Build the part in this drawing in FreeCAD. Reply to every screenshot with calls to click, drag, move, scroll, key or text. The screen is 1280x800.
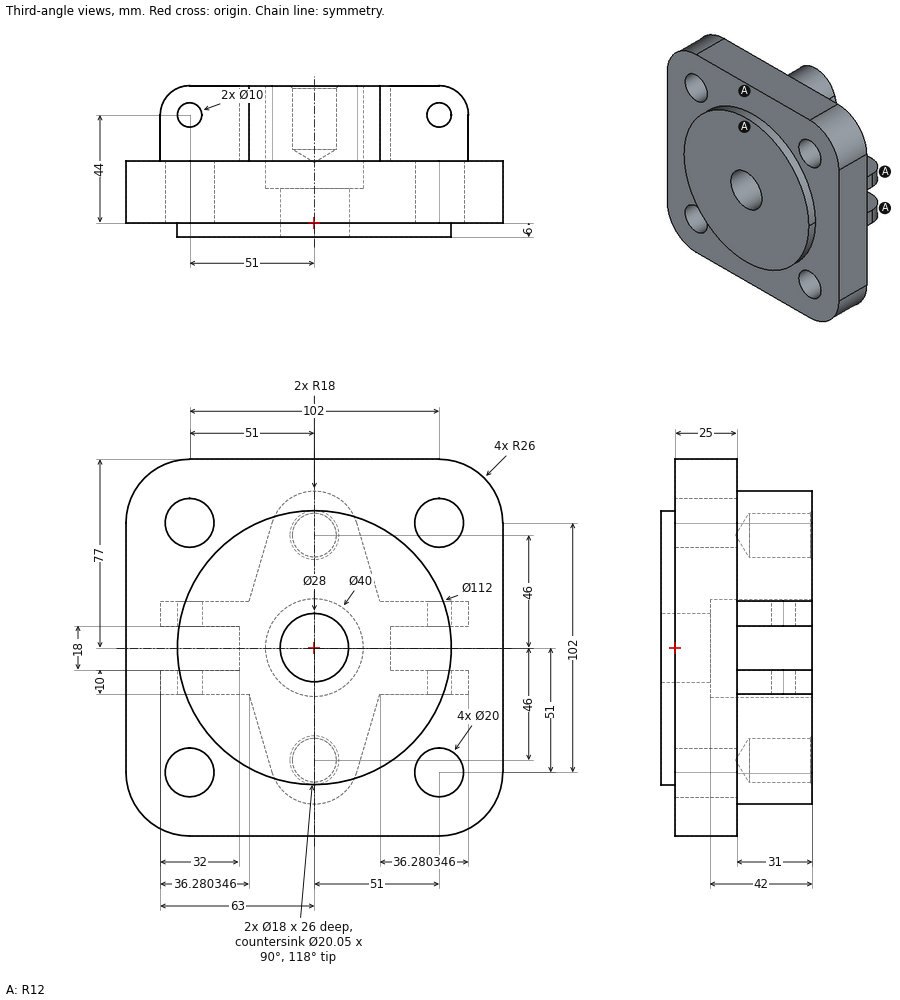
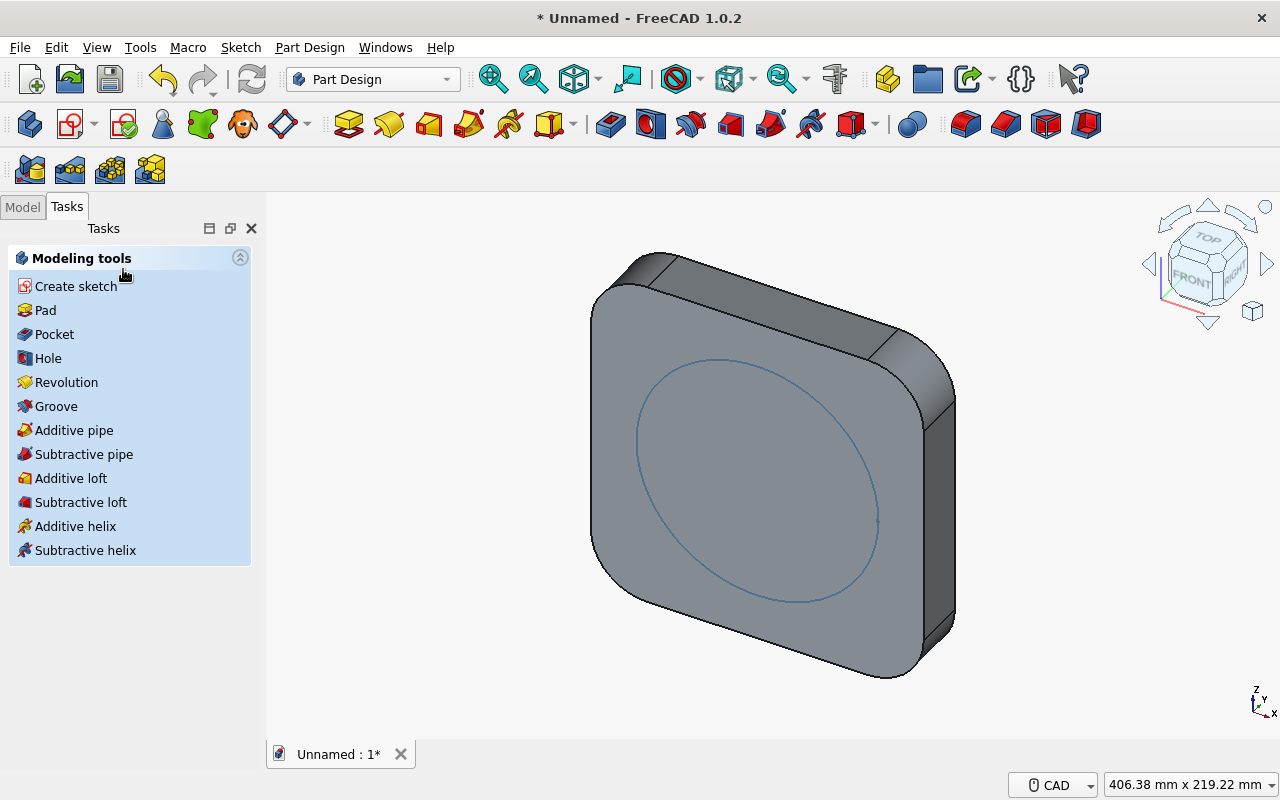
click(350, 124)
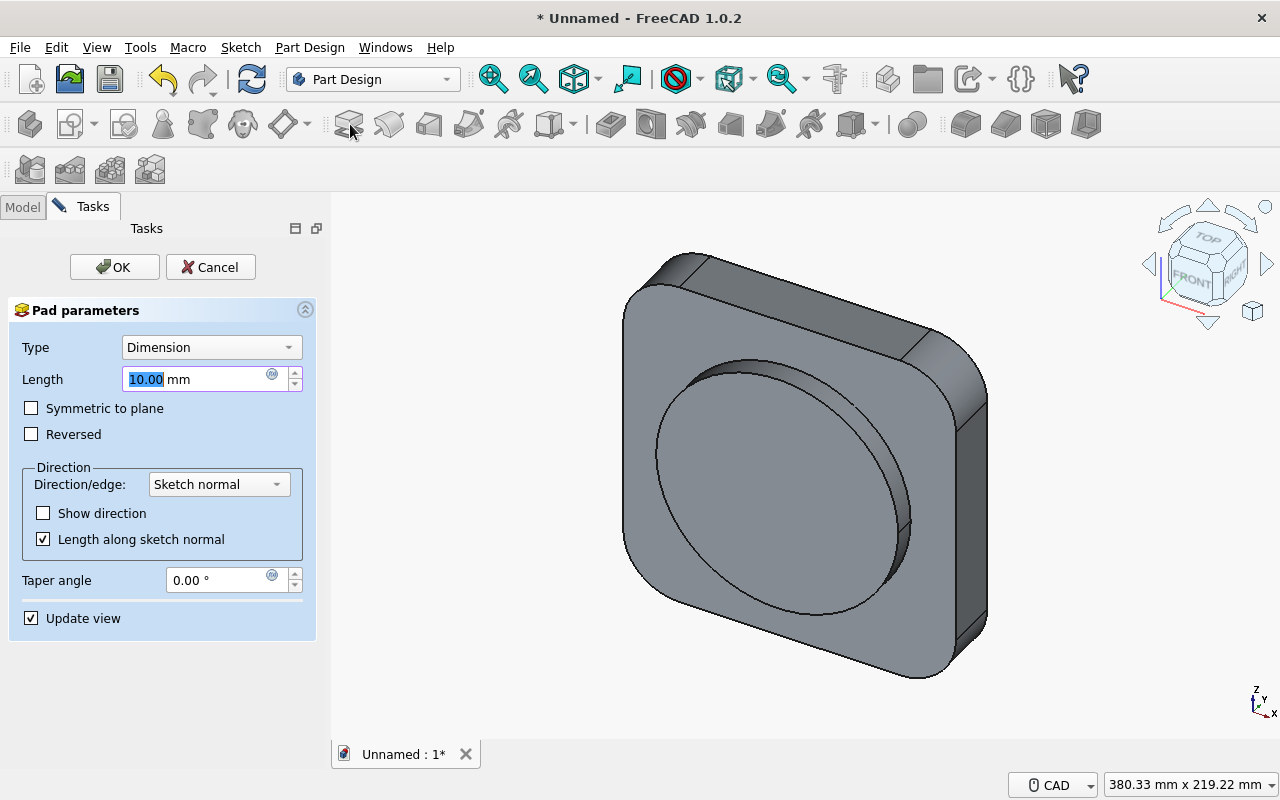
text(6)
key(Tab)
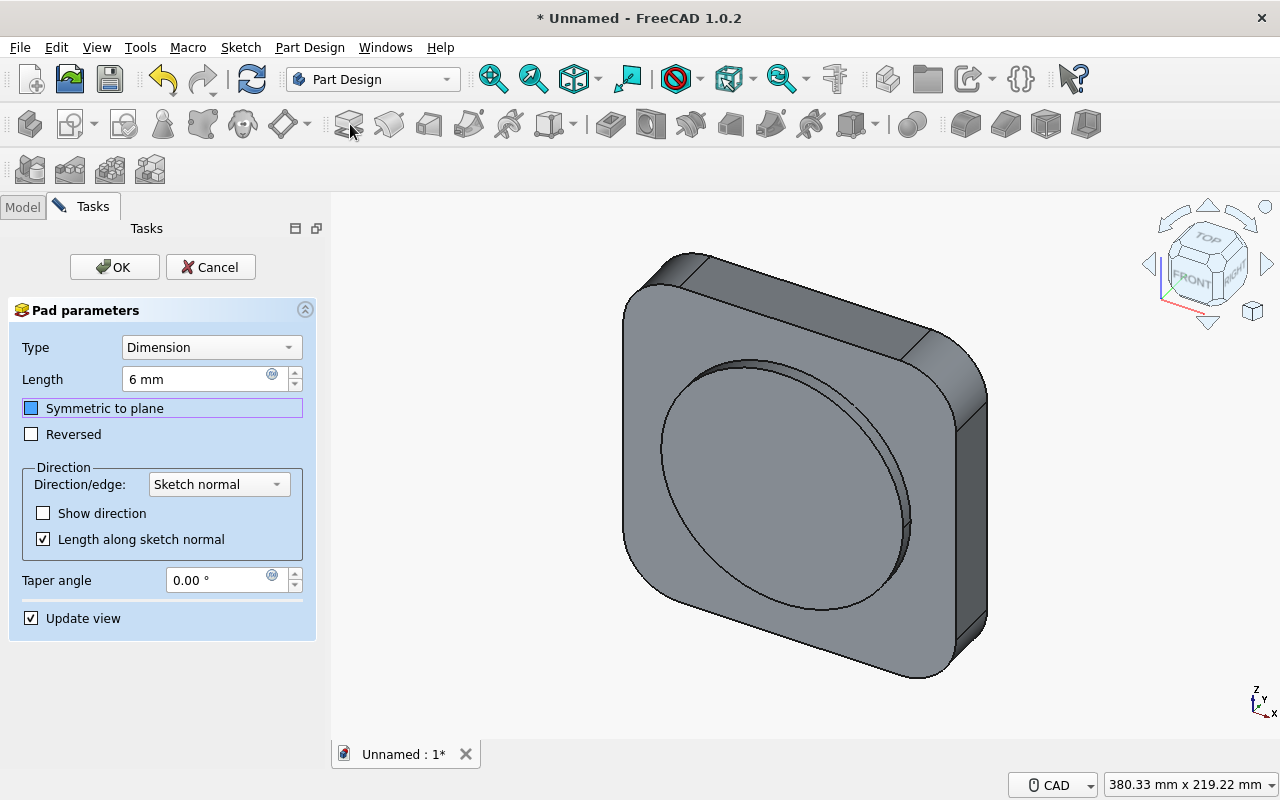
click(115, 267)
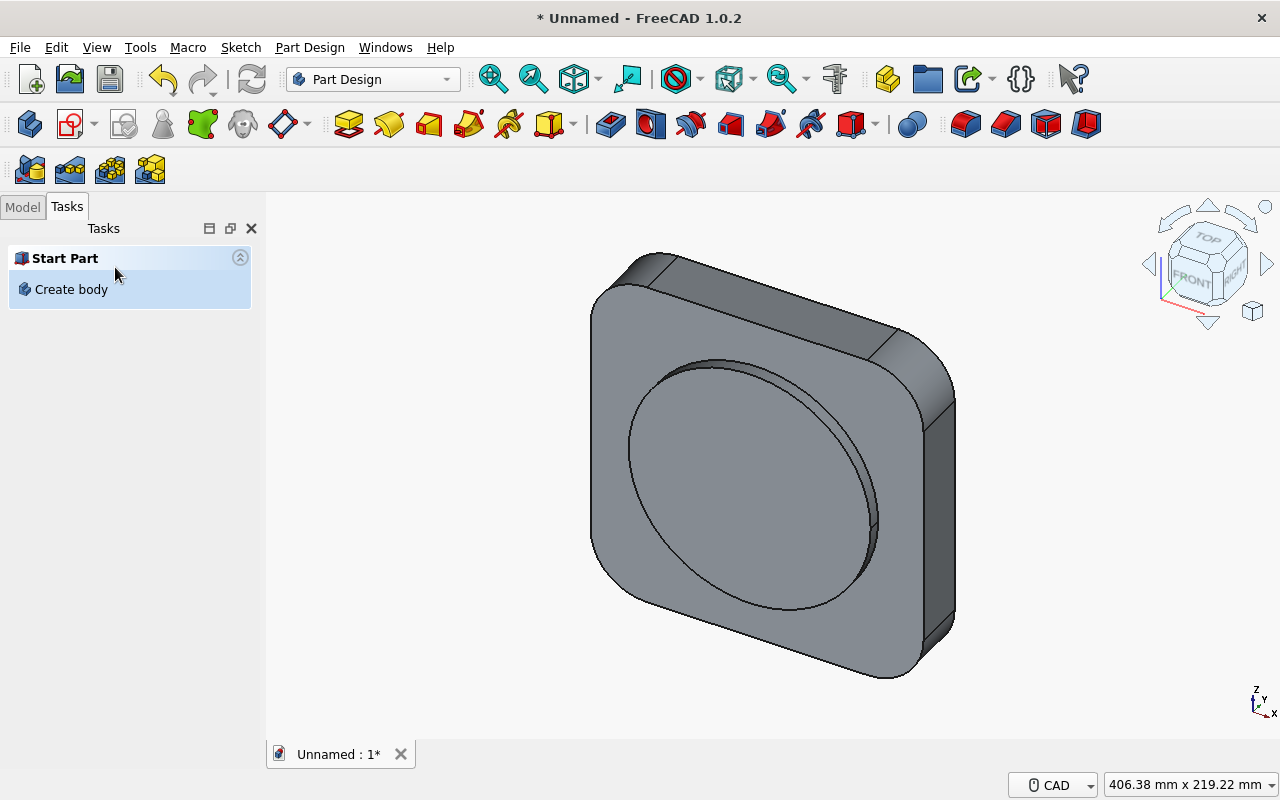
key(4)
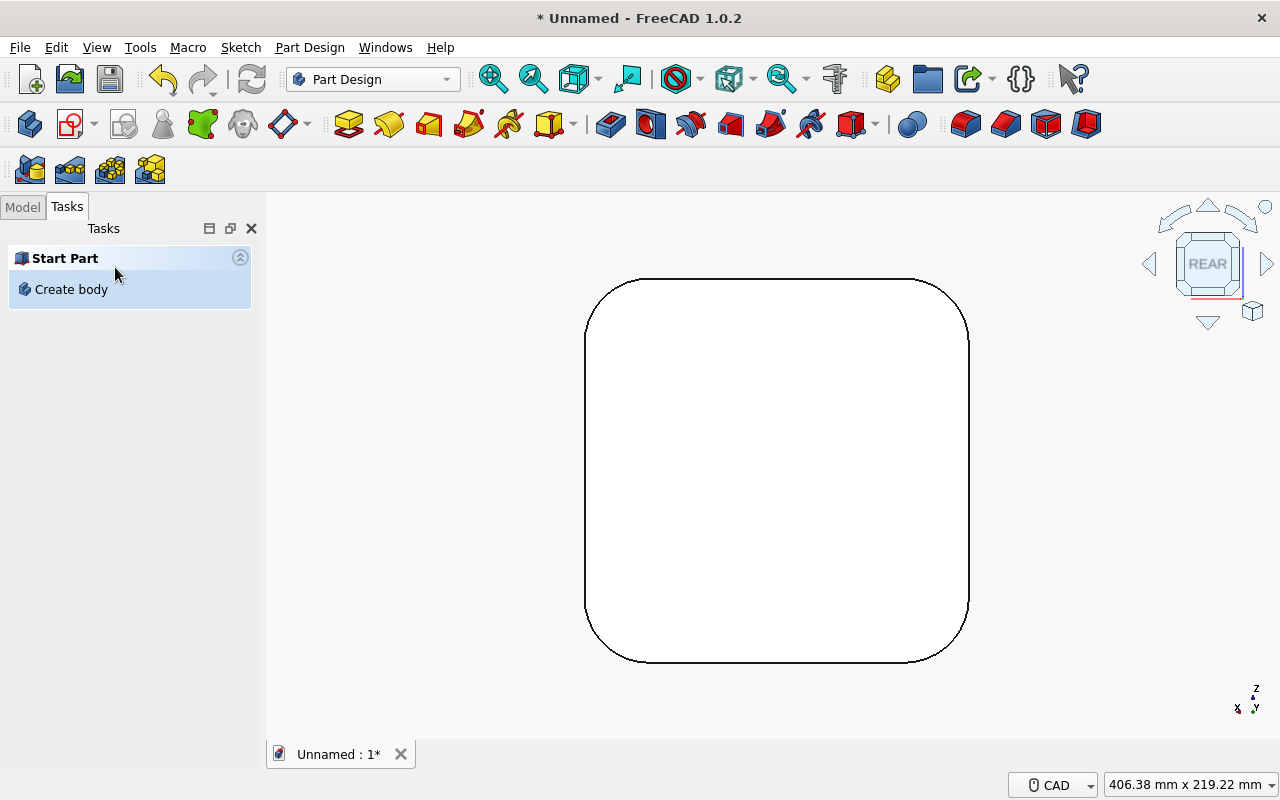
click(777, 470)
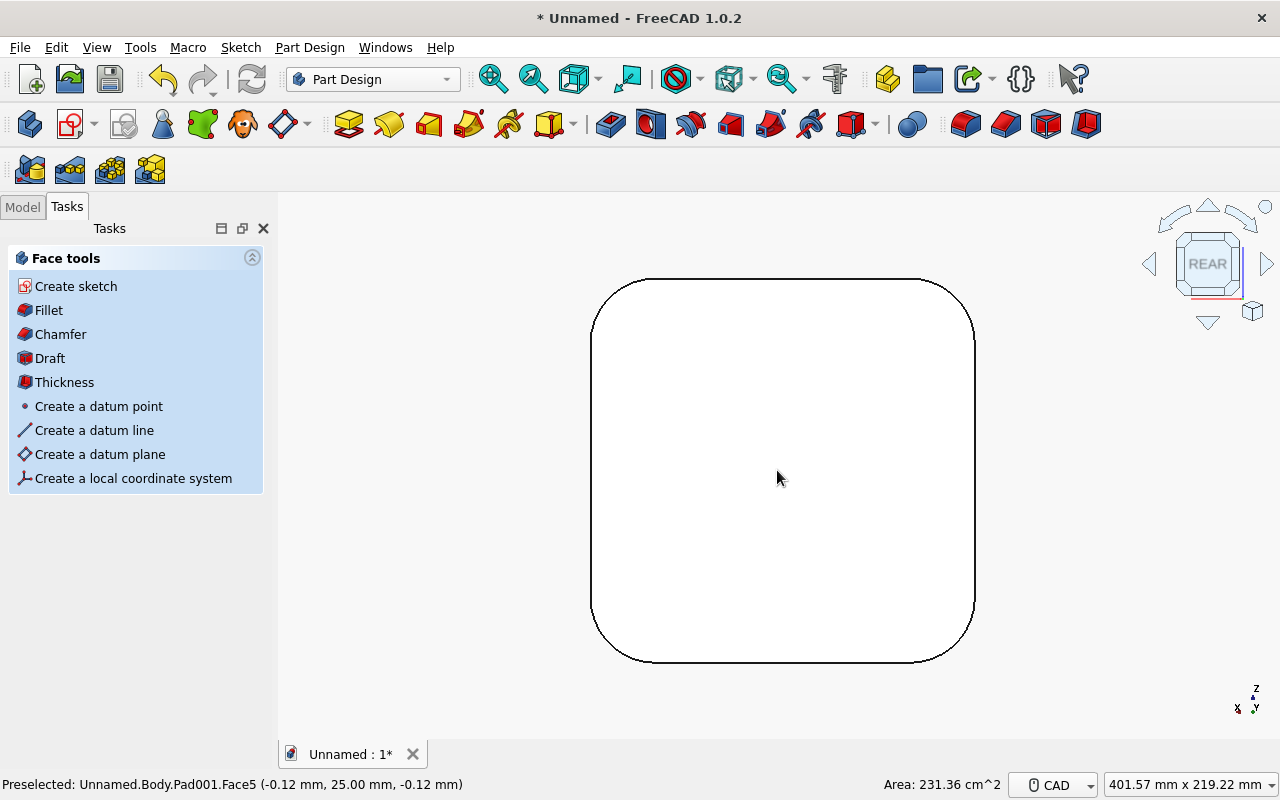
click(70, 124)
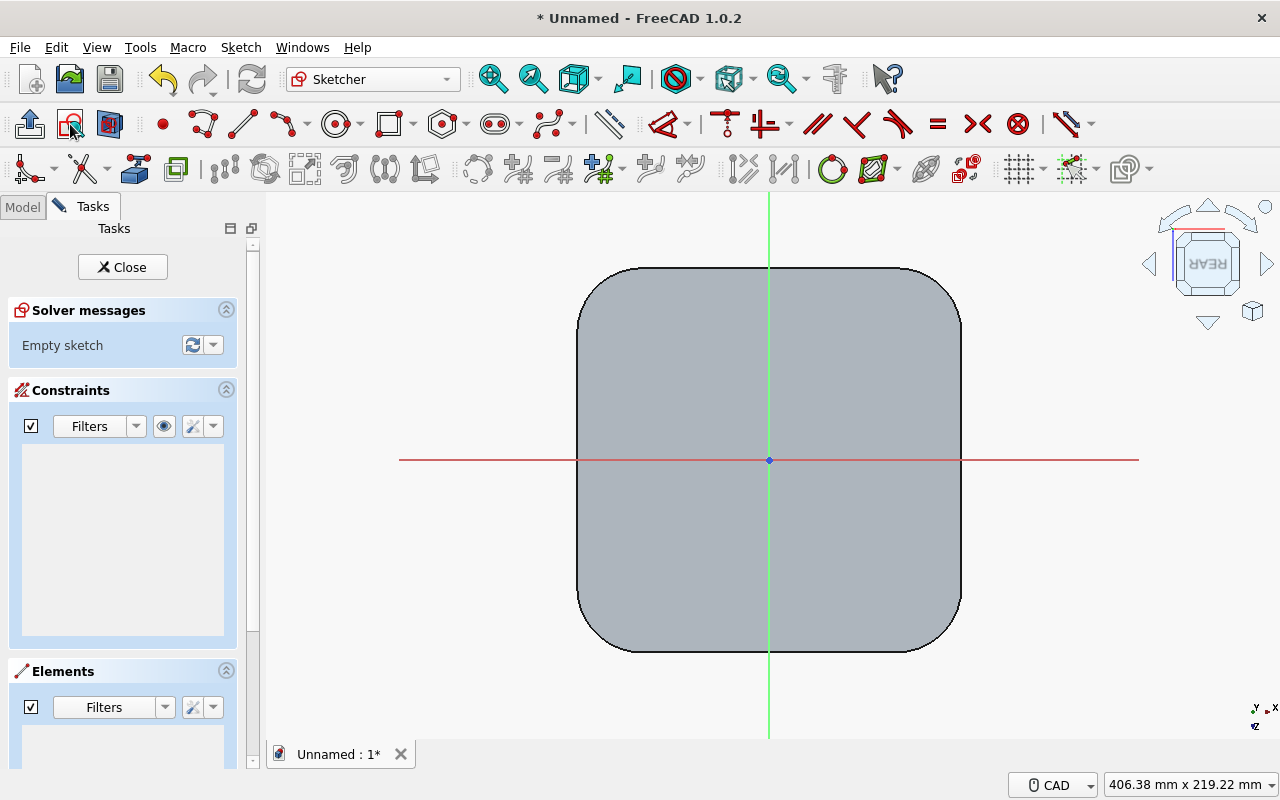
click(204, 124)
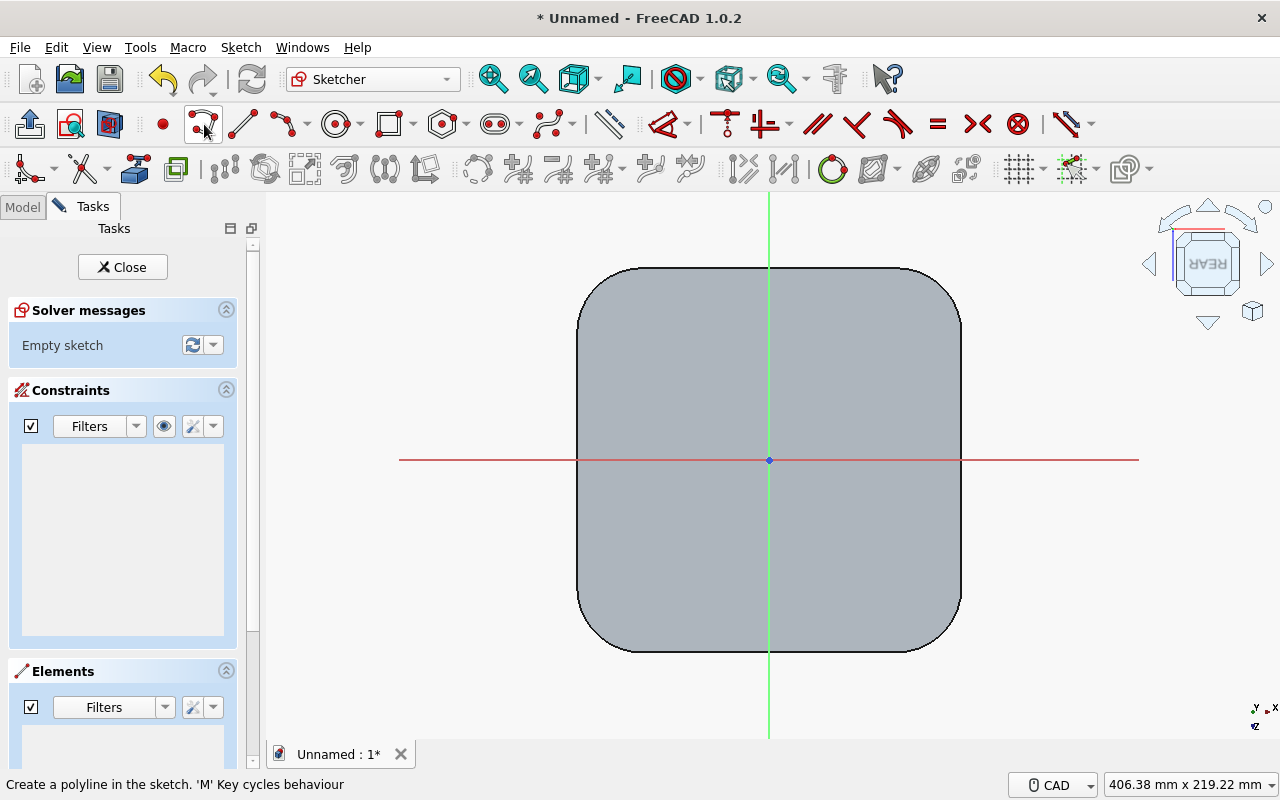
click(726, 333)
click(703, 413)
click(612, 413)
click(612, 438)
click(692, 438)
click(692, 483)
click(612, 483)
click(612, 508)
click(703, 508)
click(726, 588)
right_click(726, 588)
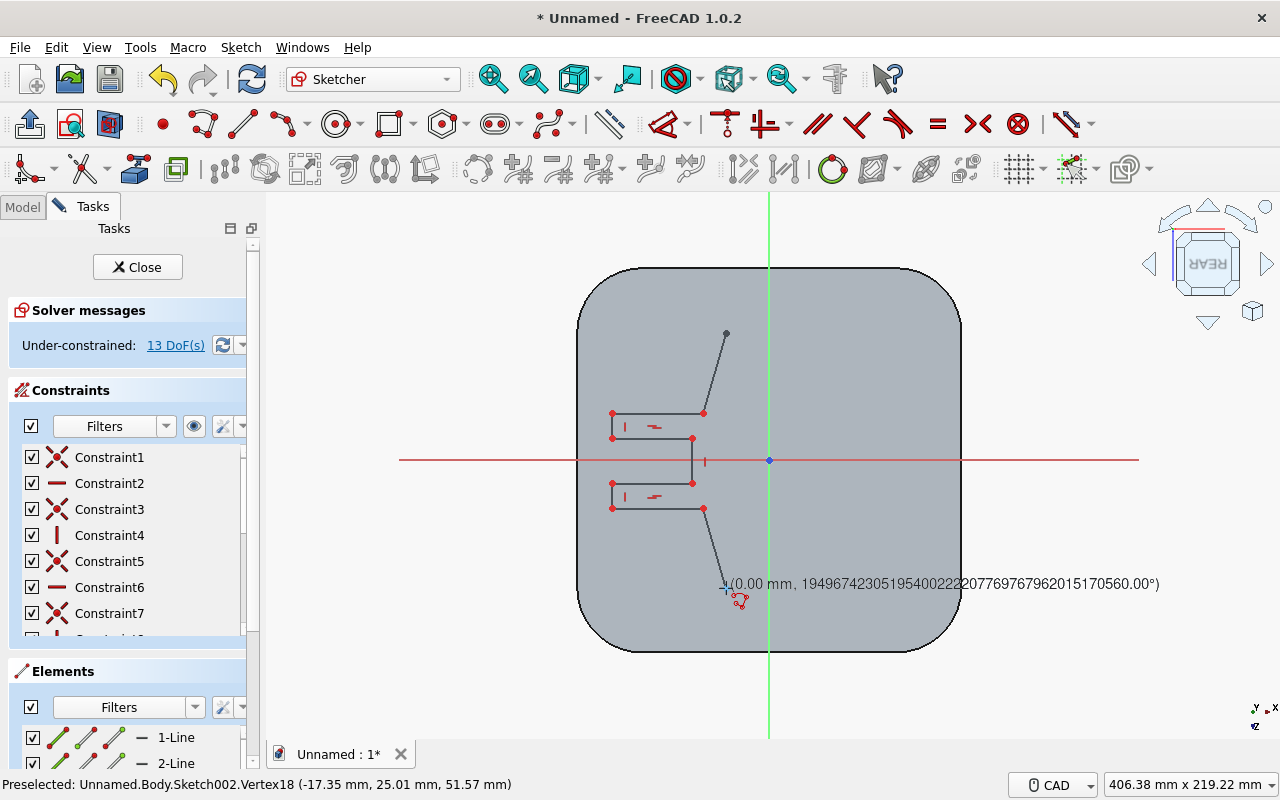
click(812, 588)
click(836, 508)
click(926, 508)
click(926, 483)
click(847, 483)
click(847, 438)
click(926, 438)
click(926, 413)
click(836, 413)
click(812, 333)
right_click(812, 333)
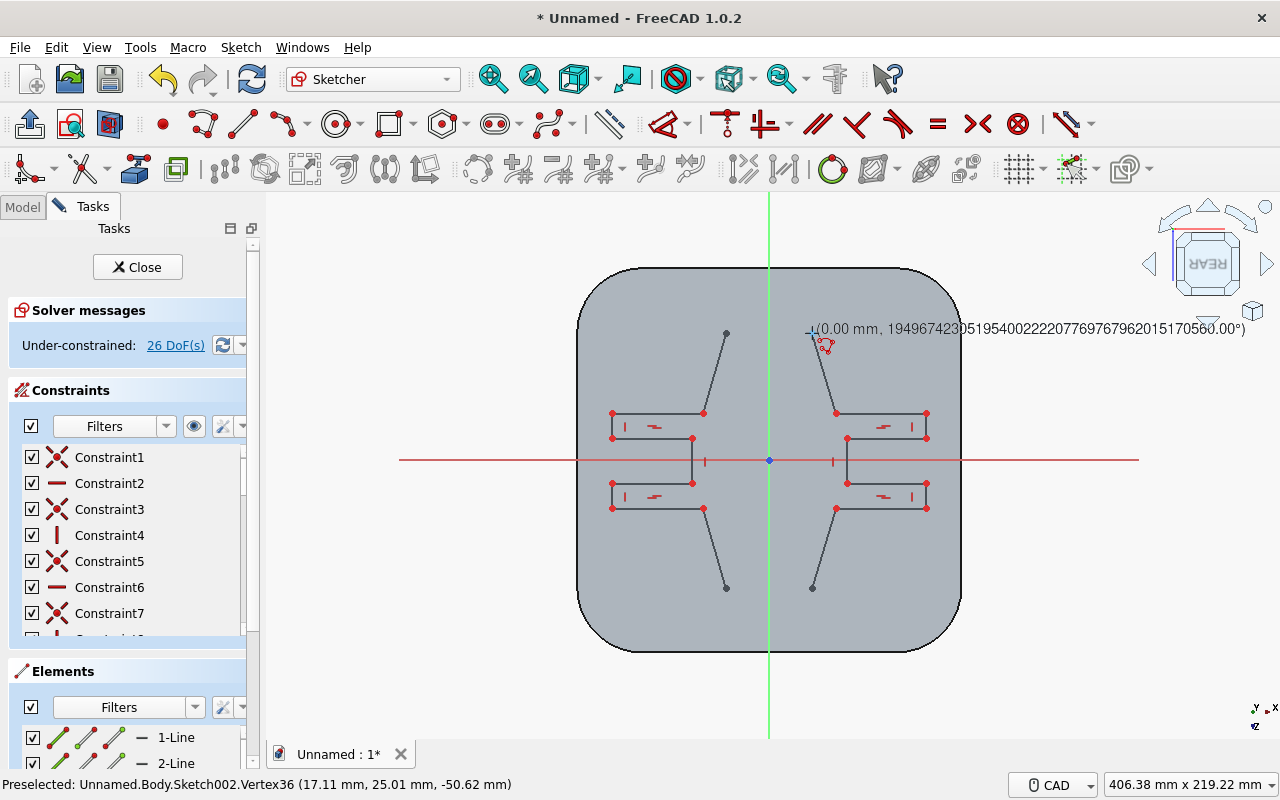
click(284, 124)